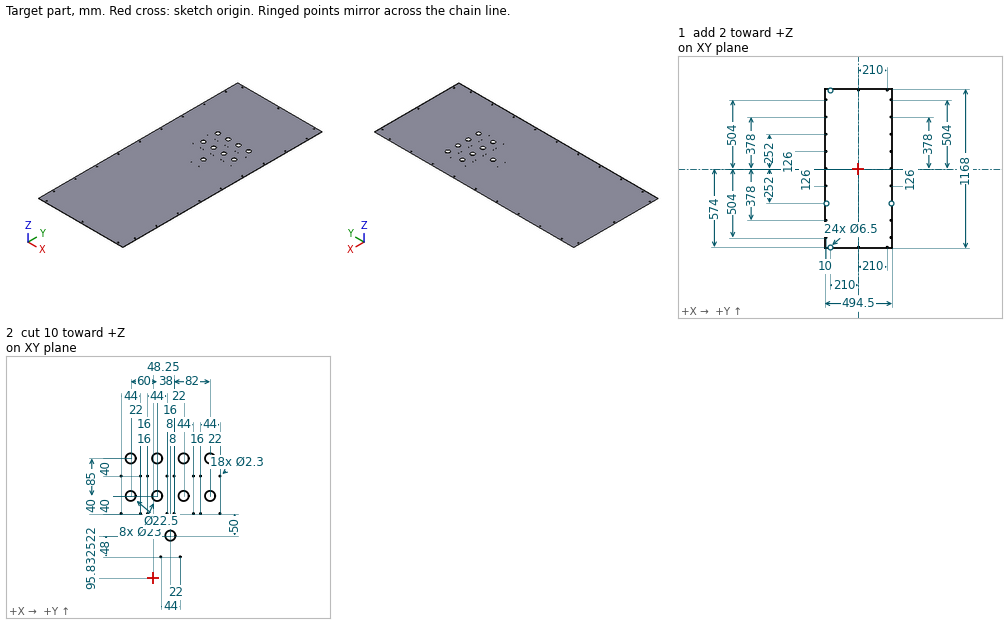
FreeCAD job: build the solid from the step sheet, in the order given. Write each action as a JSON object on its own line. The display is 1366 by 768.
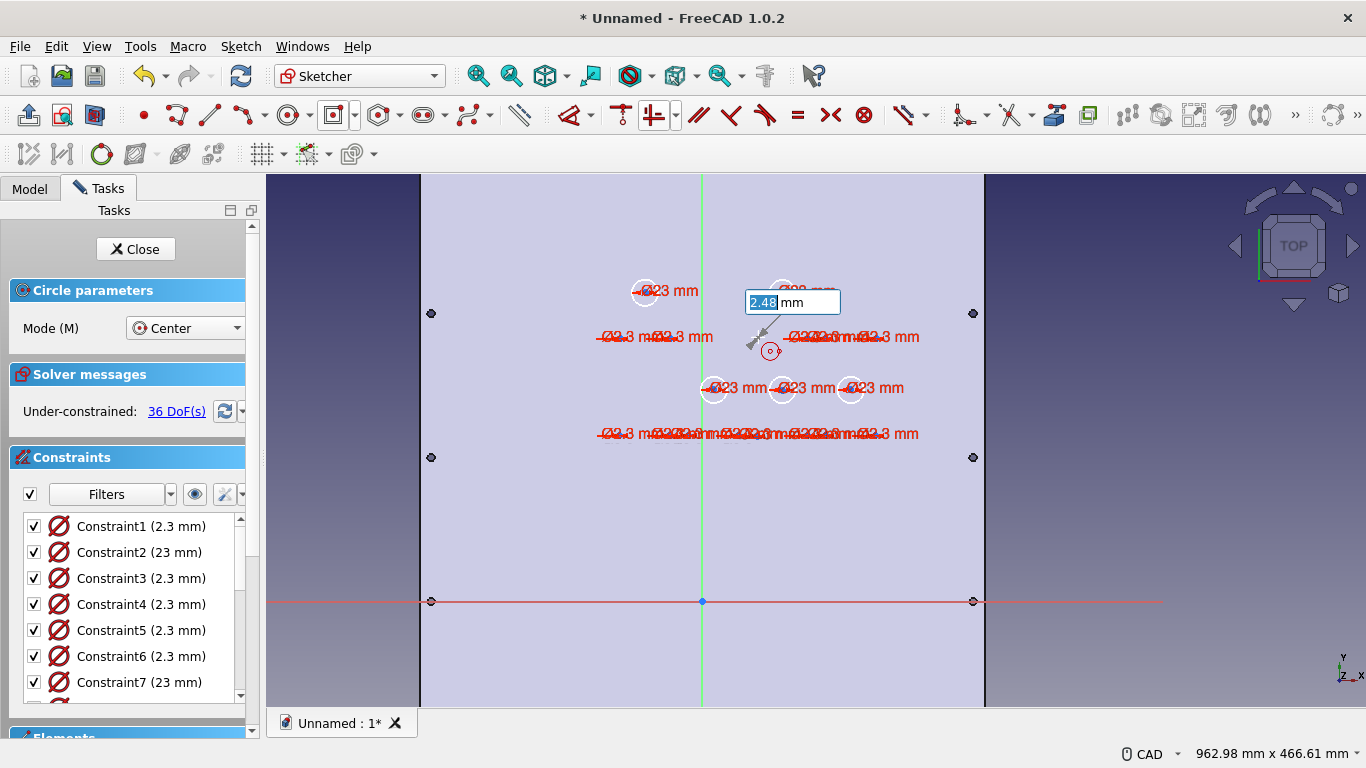
{"action": "type", "text": "2.3"}
{"action": "key", "text": "Return"}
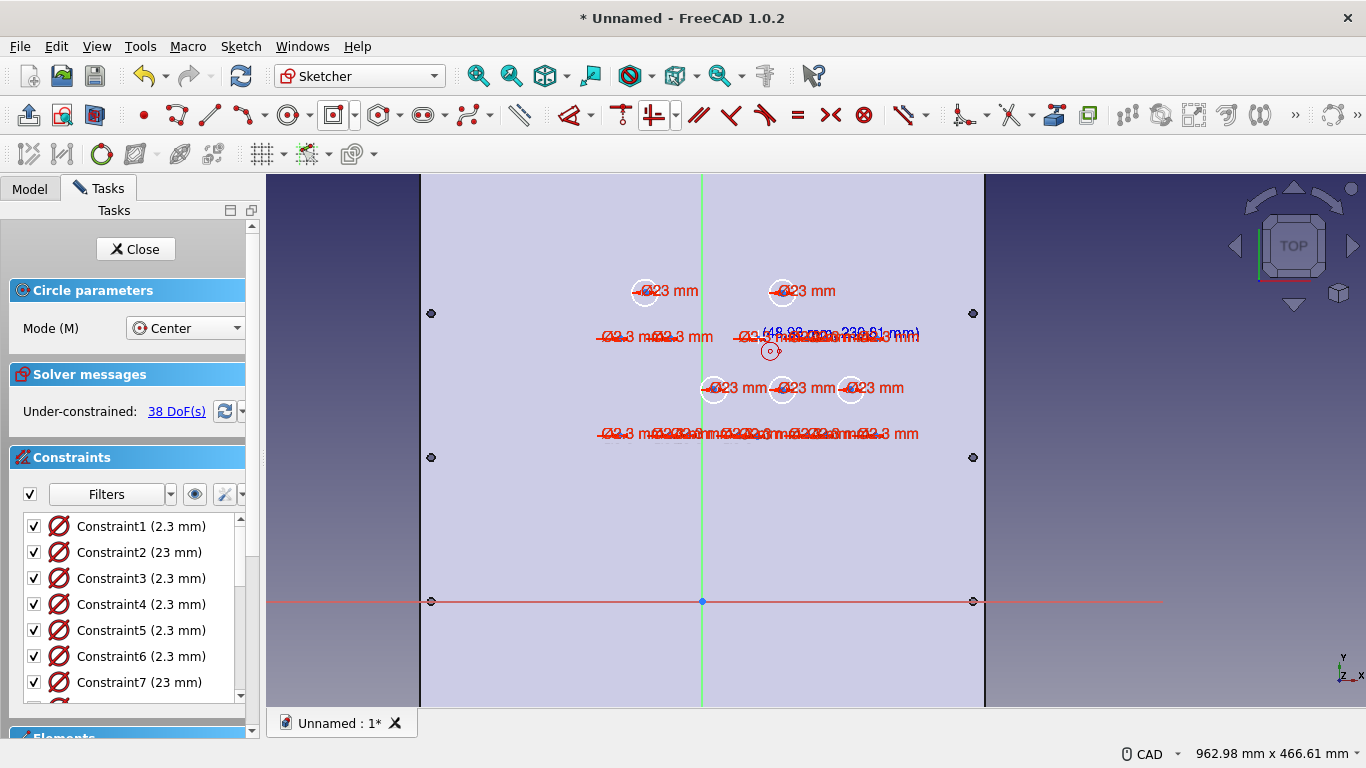
{"action": "scroll", "coordinate": [714, 292], "scroll_direction": "up", "scroll_amount": 3}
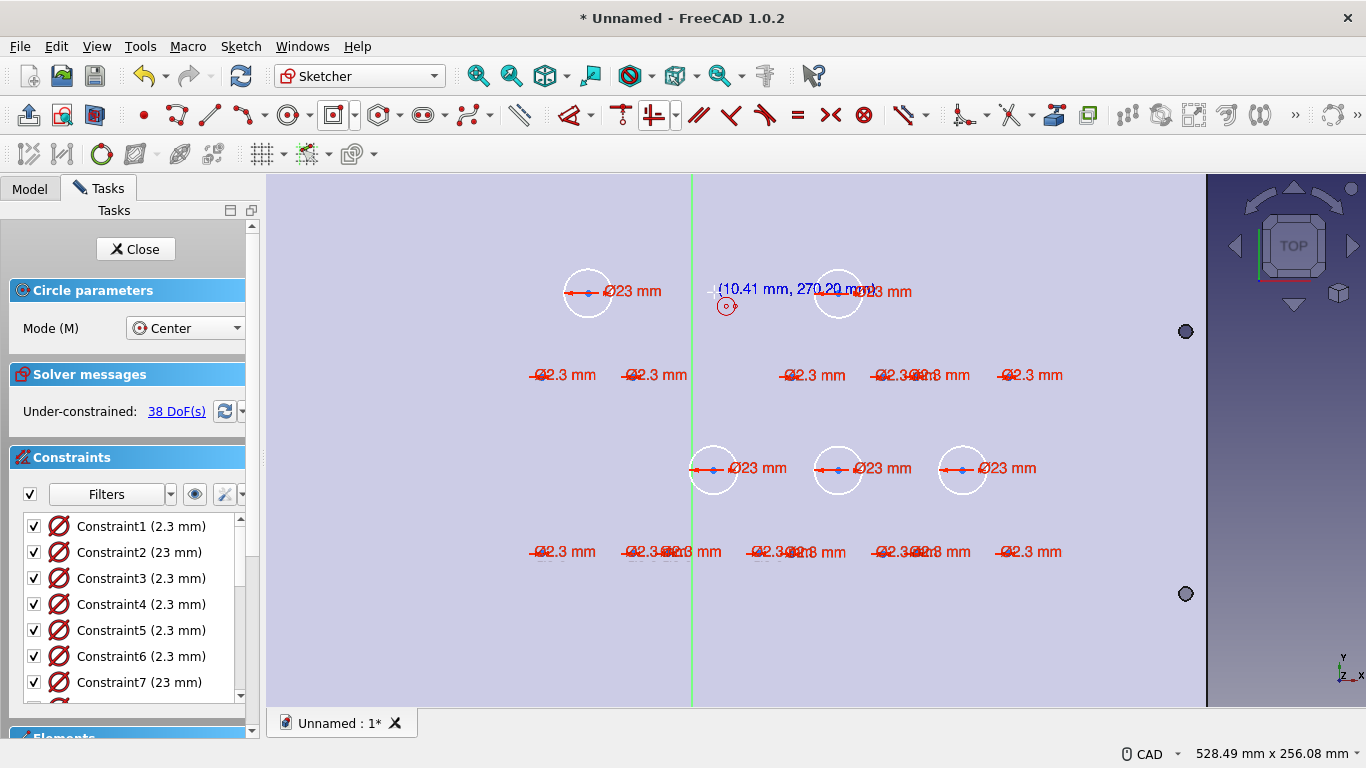
{"action": "left_click", "coordinate": [713, 292]}
{"action": "mouse_move", "coordinate": [730, 275]}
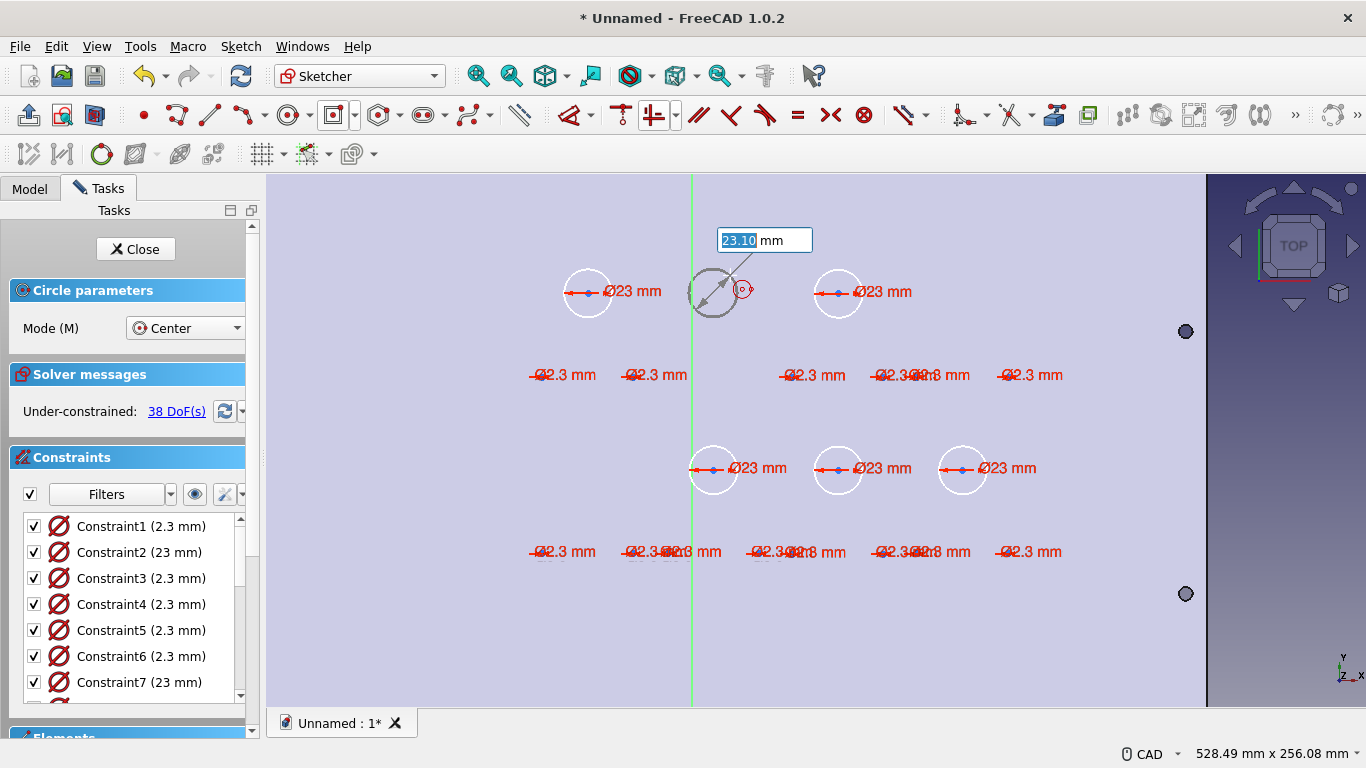
{"action": "type", "text": "23"}
{"action": "key", "text": "Return"}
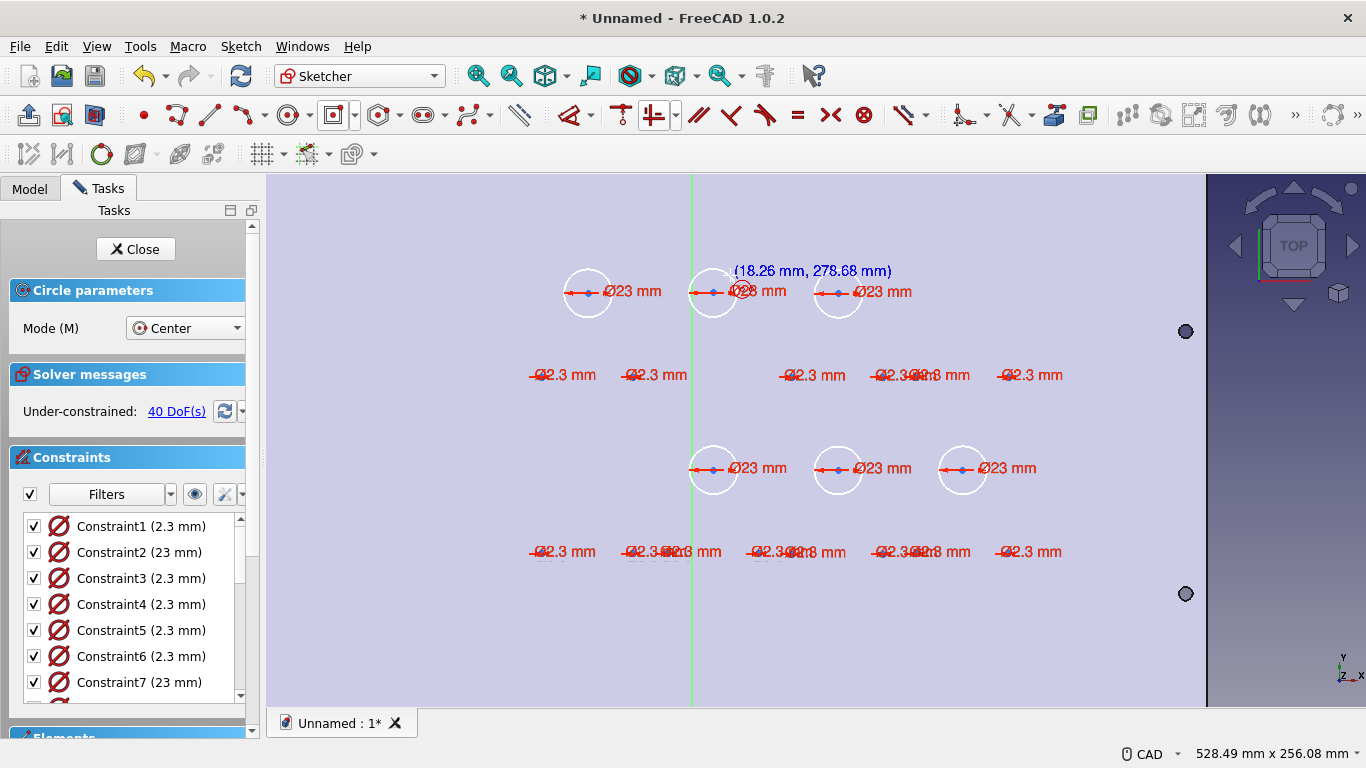
{"action": "scroll", "coordinate": [759, 376], "scroll_direction": "up", "scroll_amount": 12}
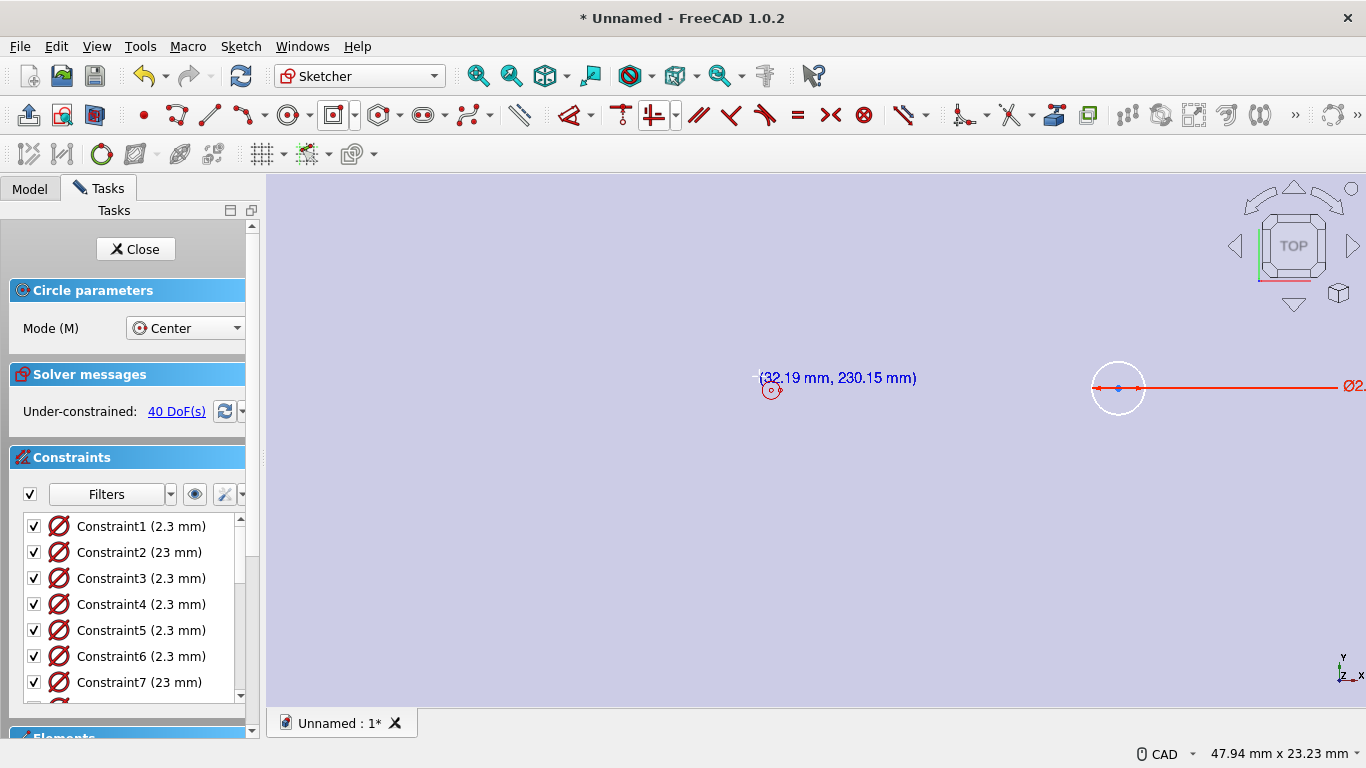
{"action": "scroll", "coordinate": [737, 337], "scroll_direction": "down", "scroll_amount": 15}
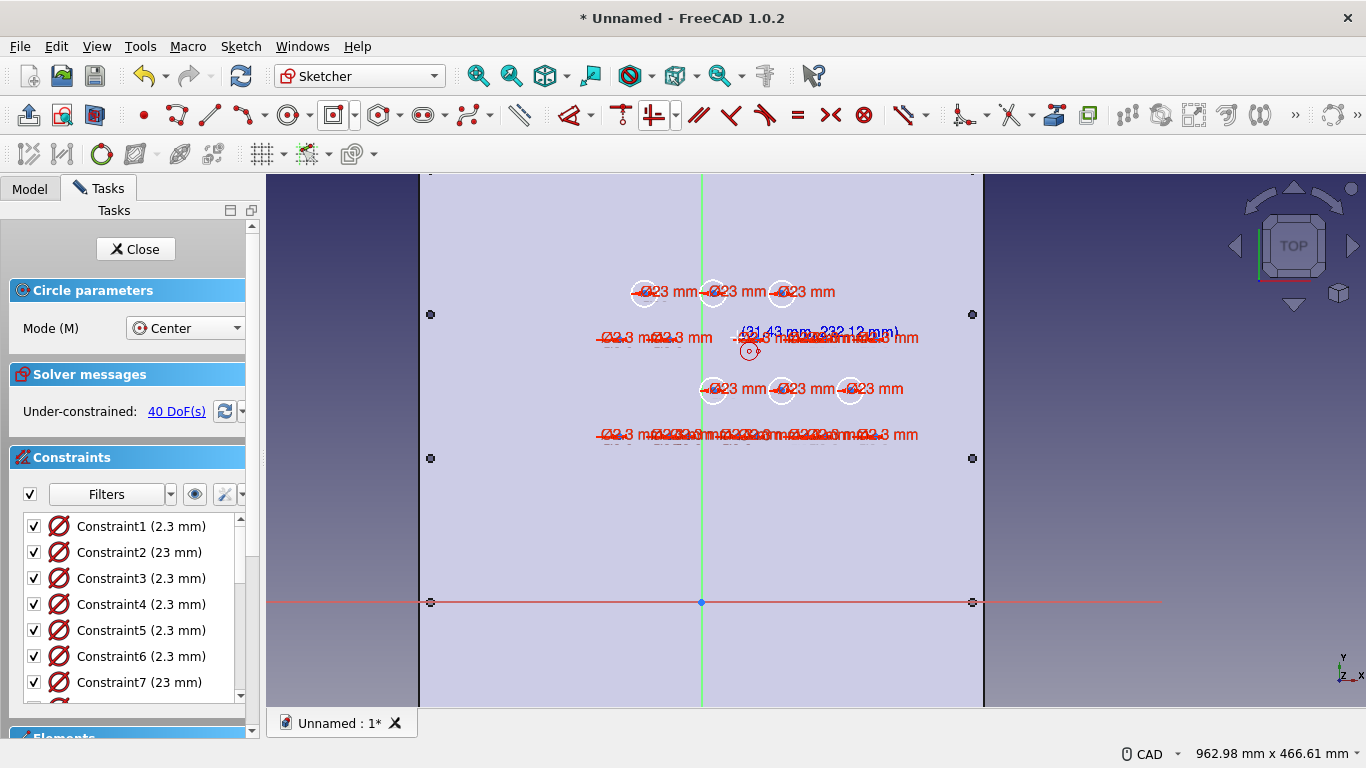
{"action": "left_click", "coordinate": [738, 339]}
{"action": "mouse_move", "coordinate": [739, 338]}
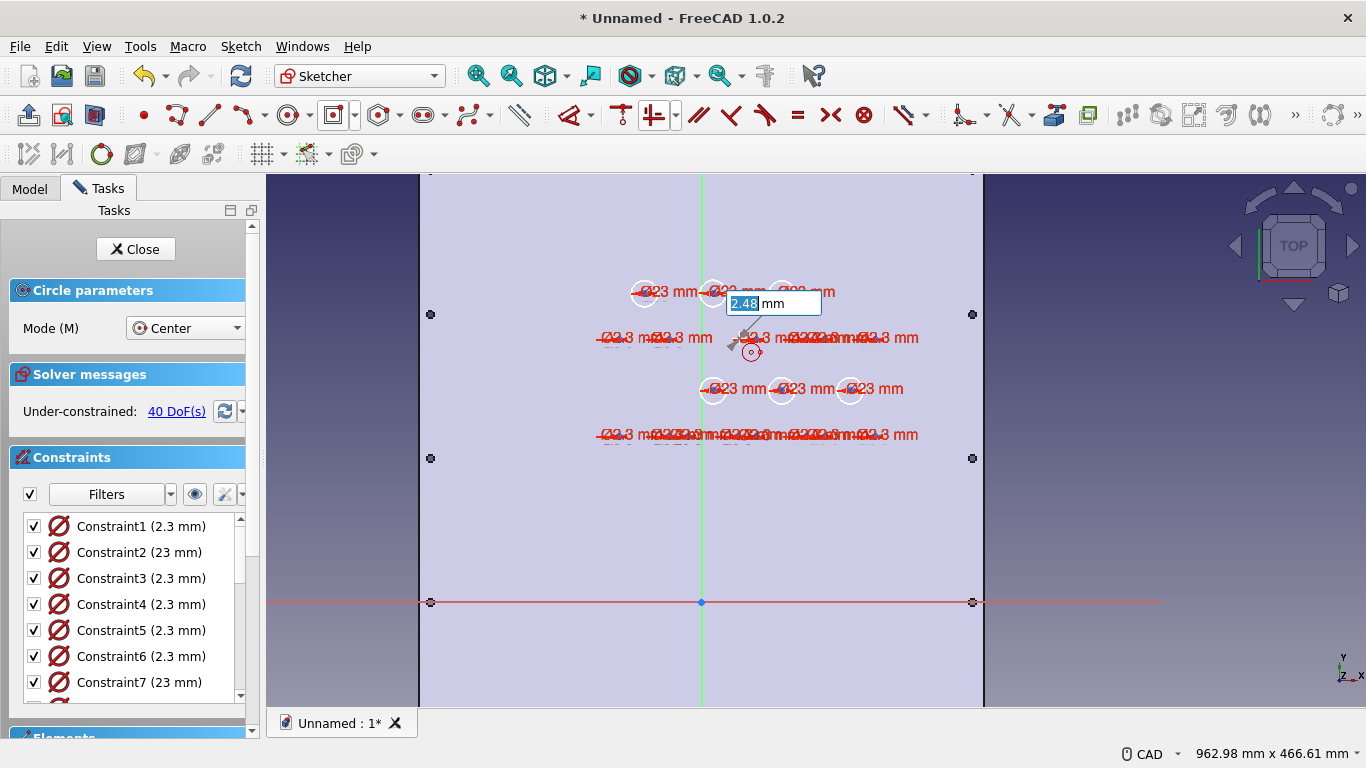
{"action": "type", "text": "2.3"}
{"action": "key", "text": "Return"}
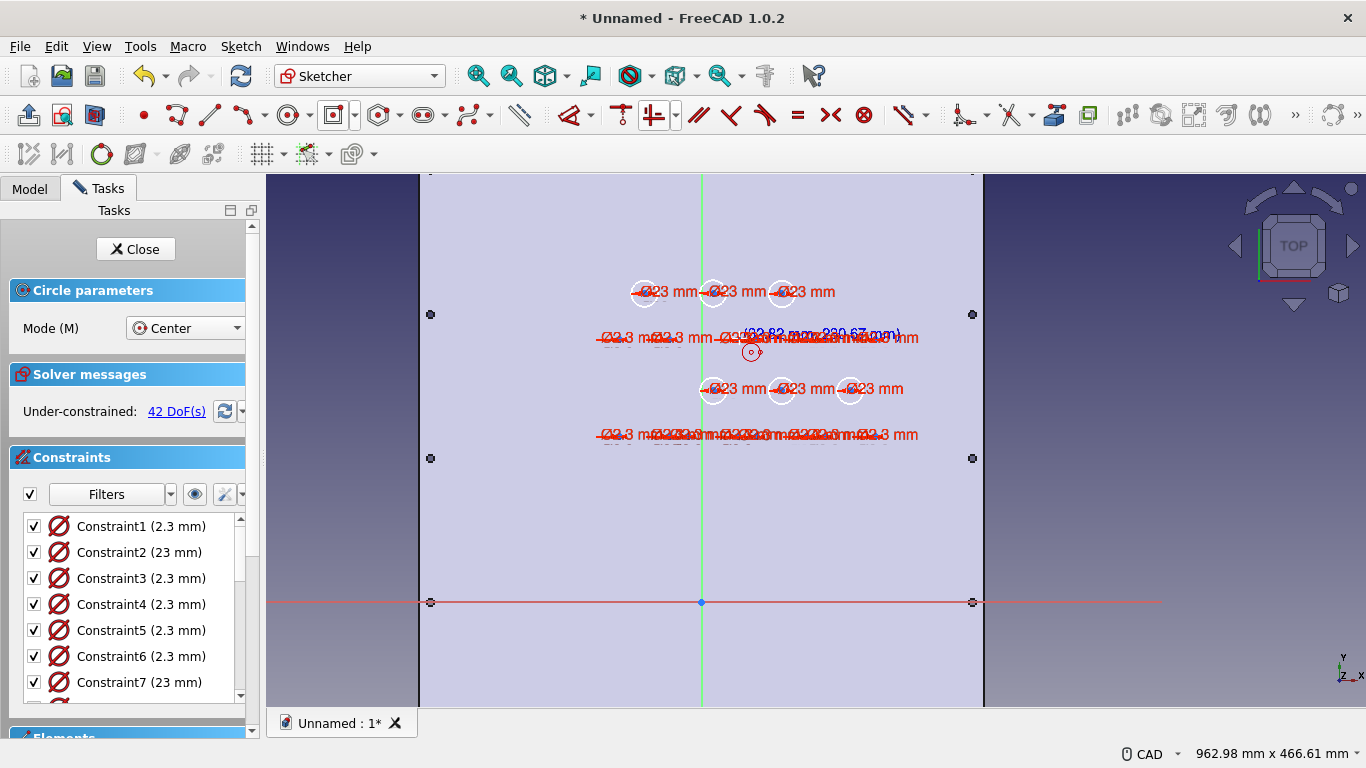
{"action": "scroll", "coordinate": [688, 339], "scroll_direction": "up", "scroll_amount": 15}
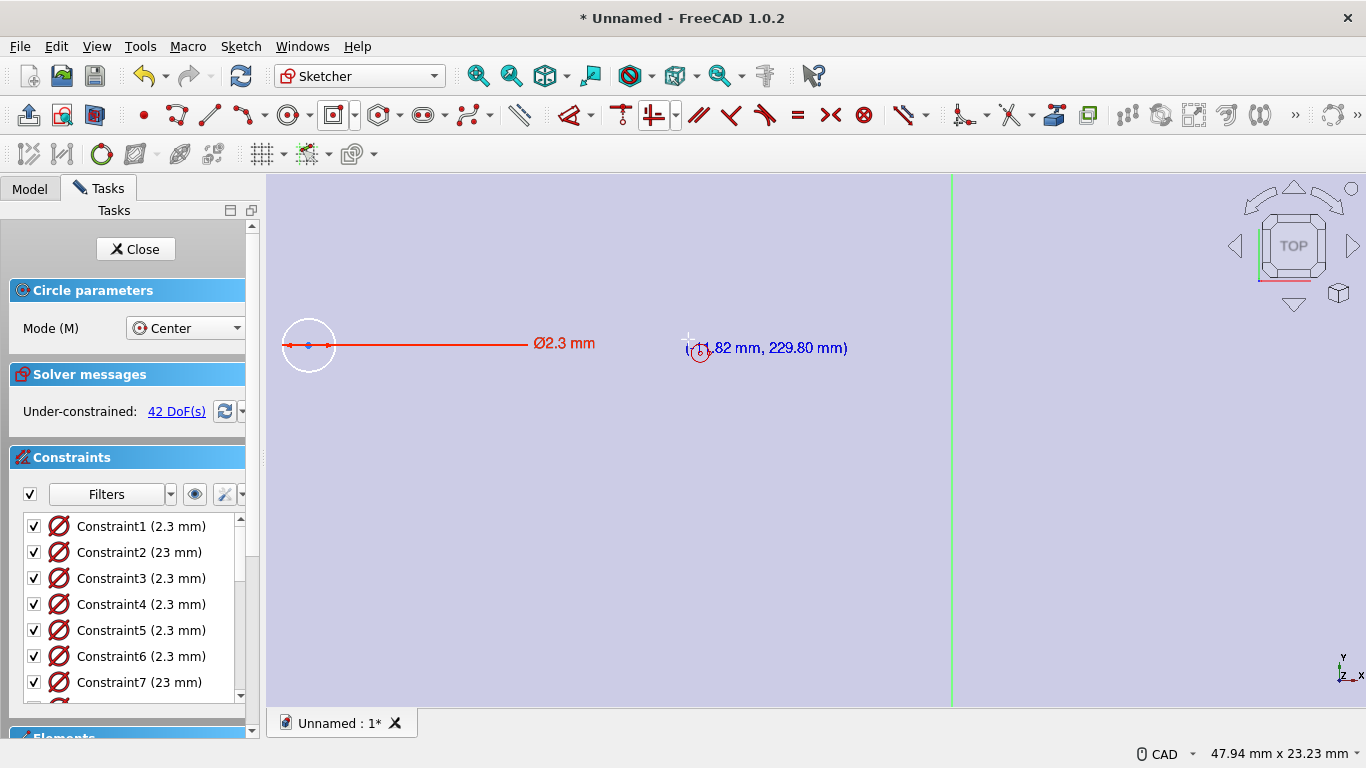
{"action": "scroll", "coordinate": [688, 339], "scroll_direction": "down", "scroll_amount": 15}